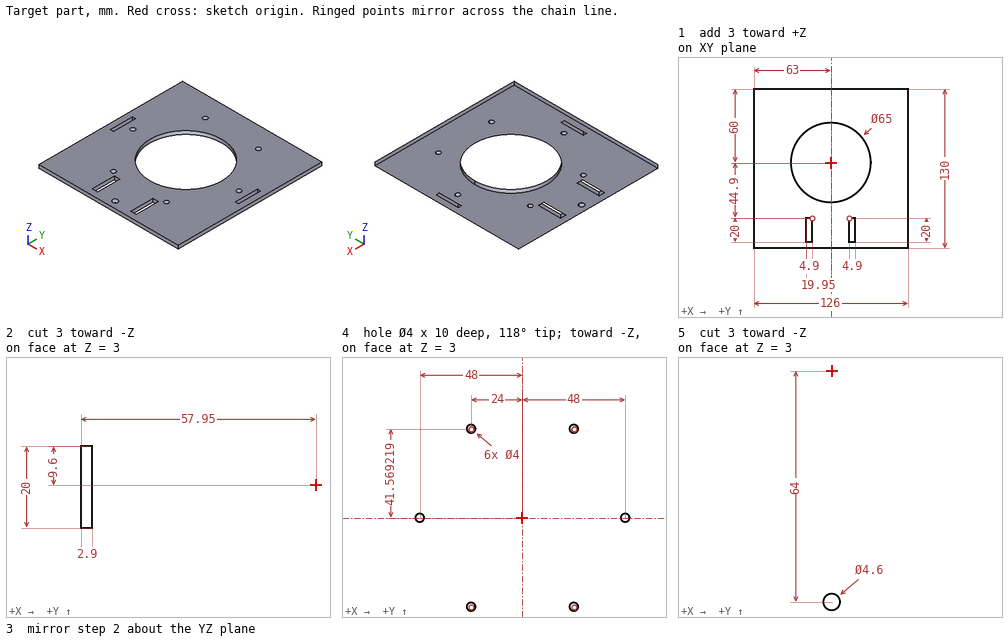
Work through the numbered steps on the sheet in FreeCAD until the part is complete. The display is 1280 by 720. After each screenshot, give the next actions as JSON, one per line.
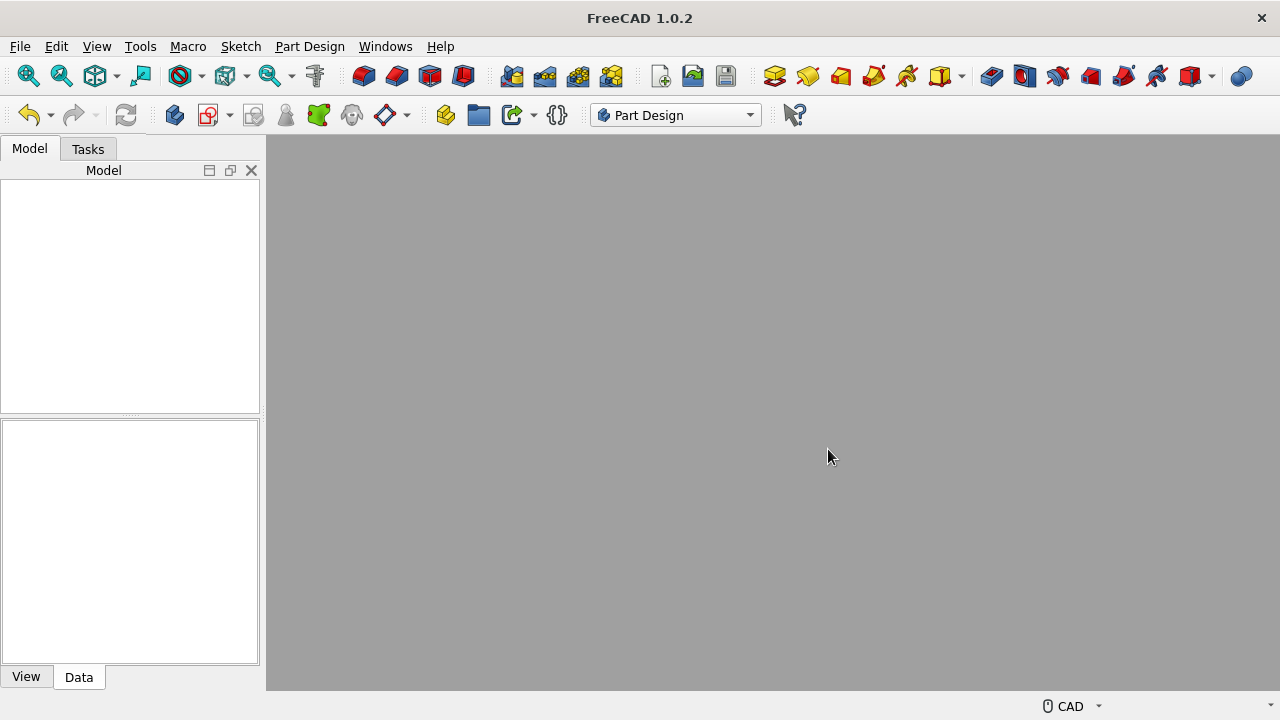
{"action": "left_click", "coordinate": [660, 76]}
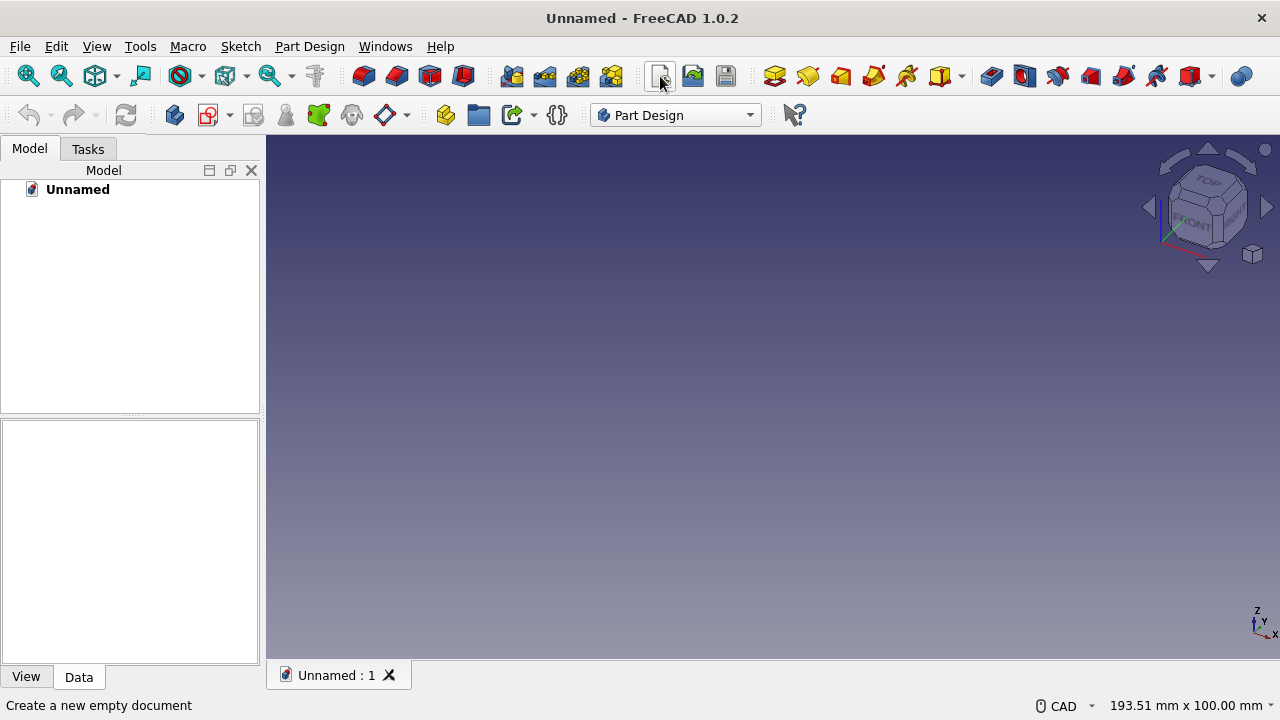
{"action": "left_click", "coordinate": [208, 116]}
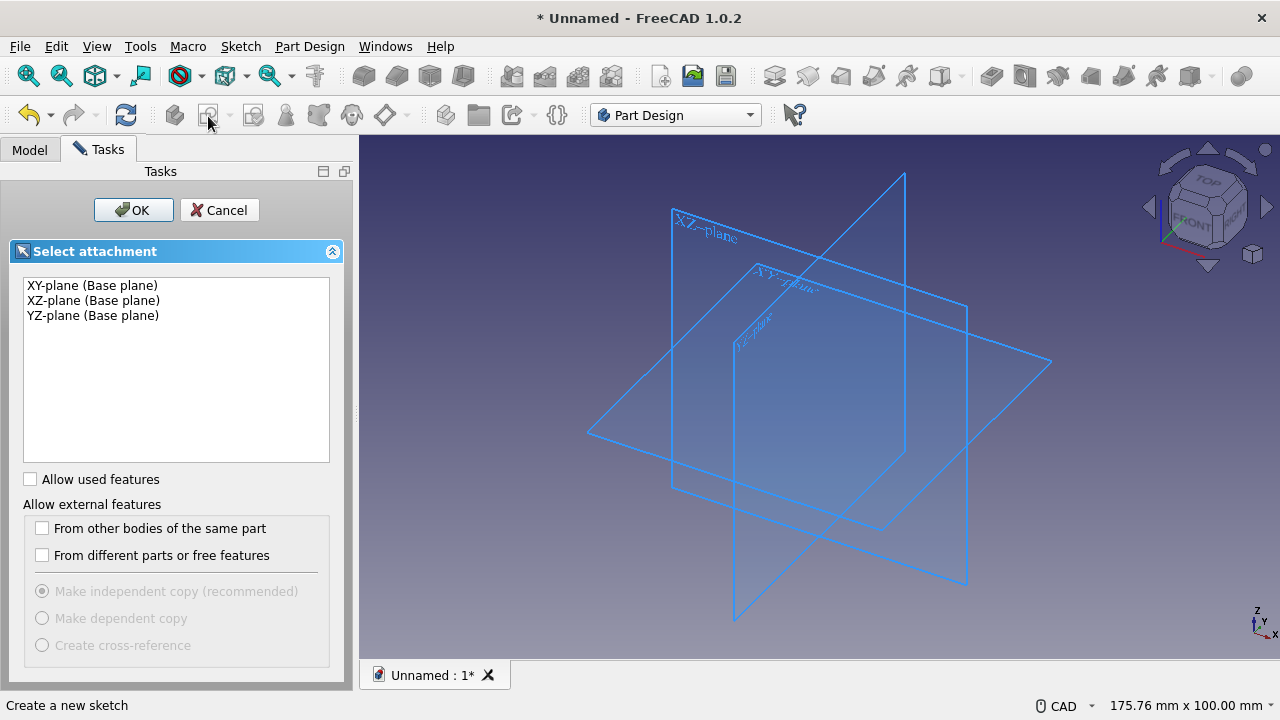
{"action": "left_click", "coordinate": [84, 286]}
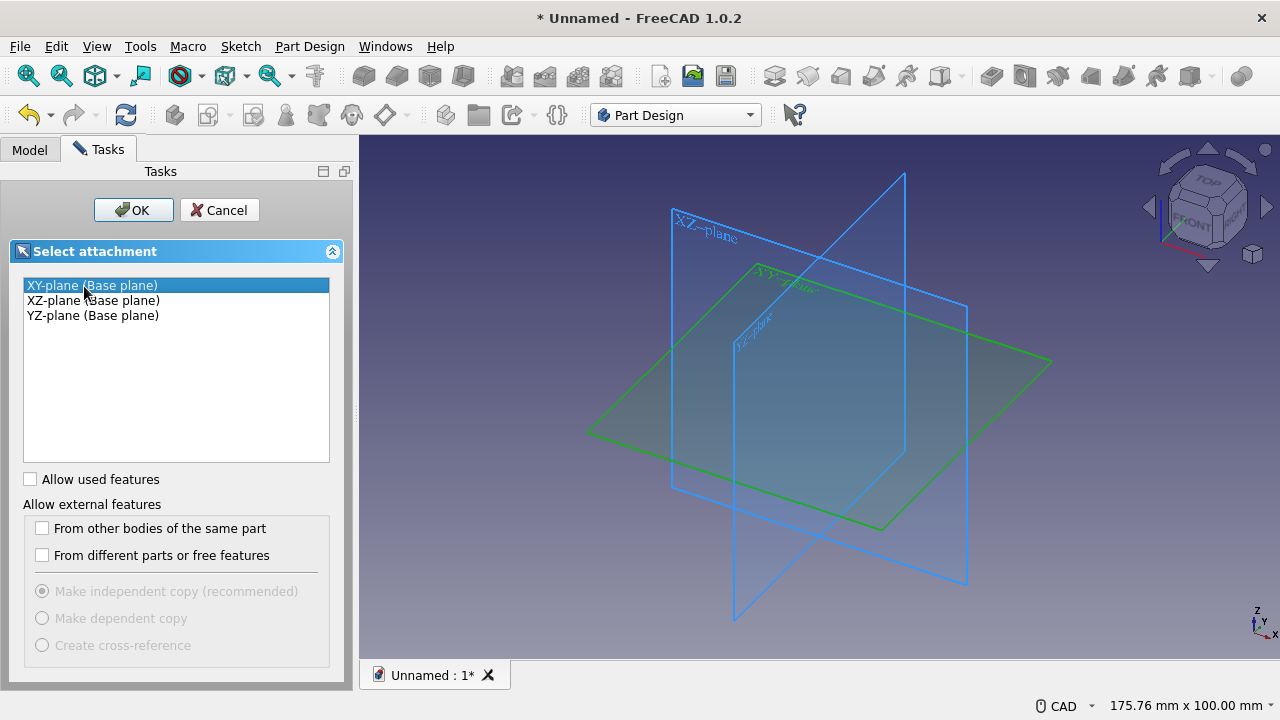
{"action": "left_click", "coordinate": [134, 210]}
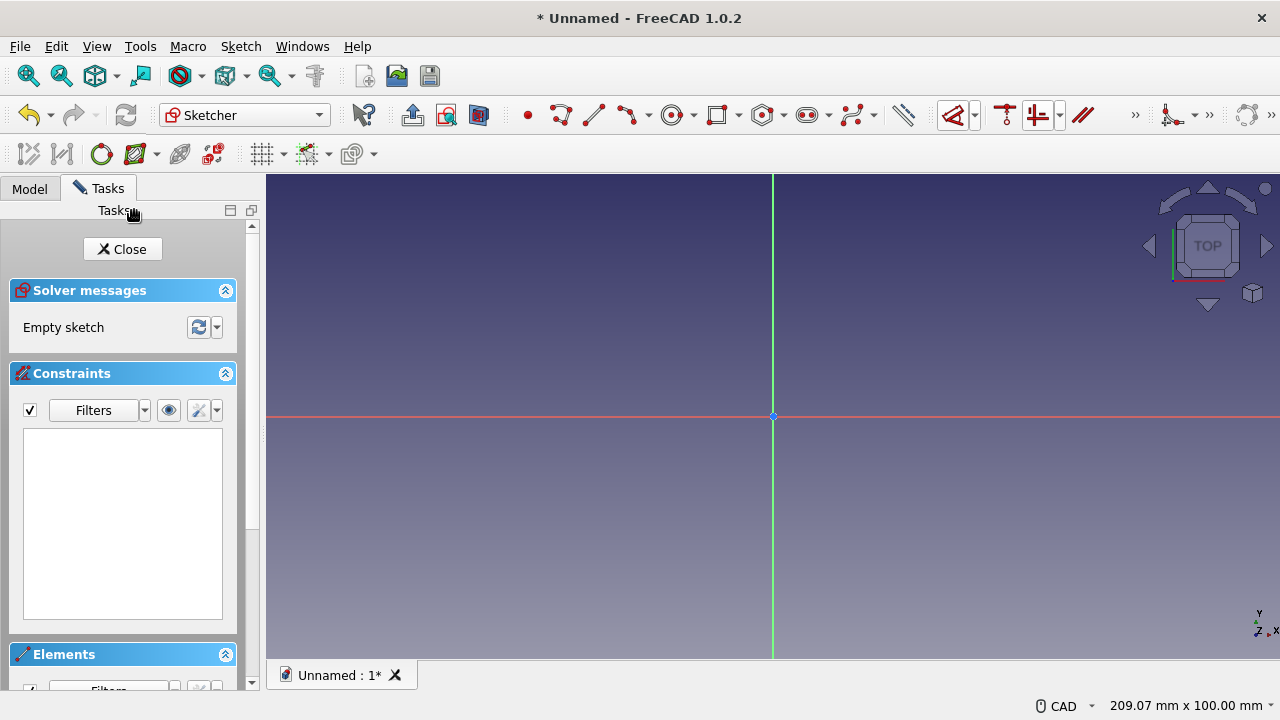
{"action": "scroll", "coordinate": [649, 397], "scroll_direction": "down", "scroll_amount": 4}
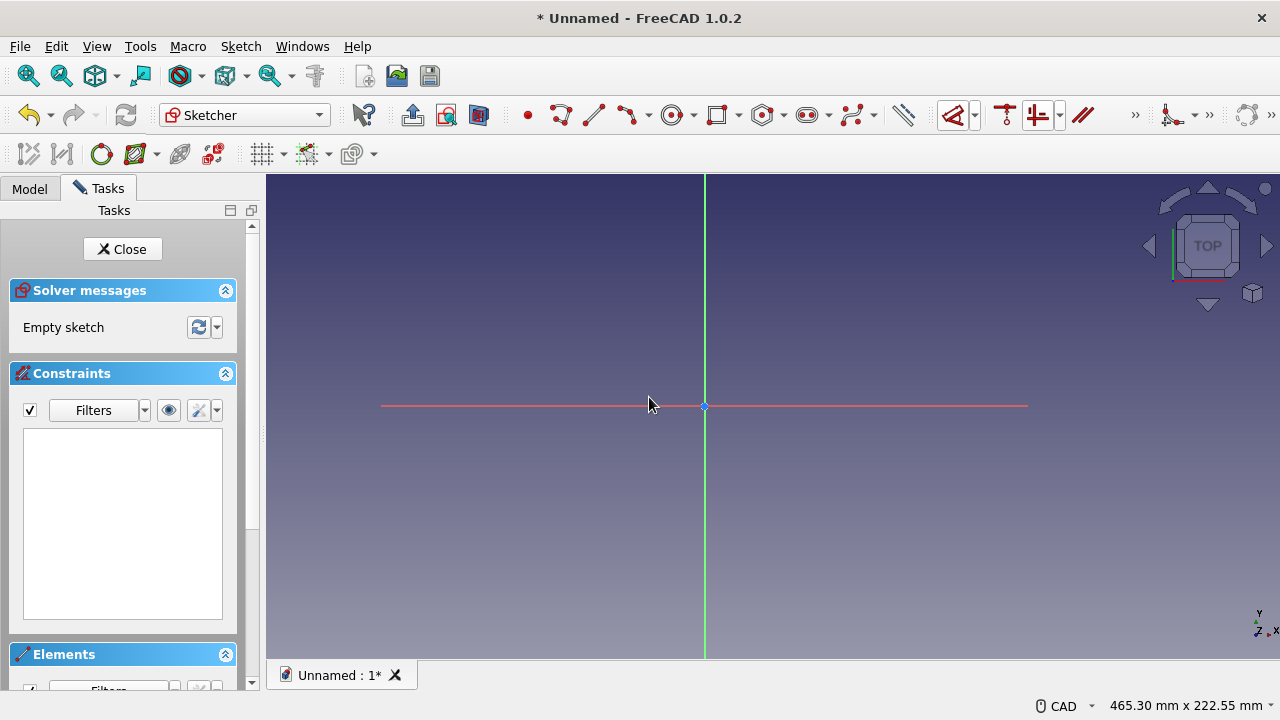
{"action": "left_click", "coordinate": [716, 116]}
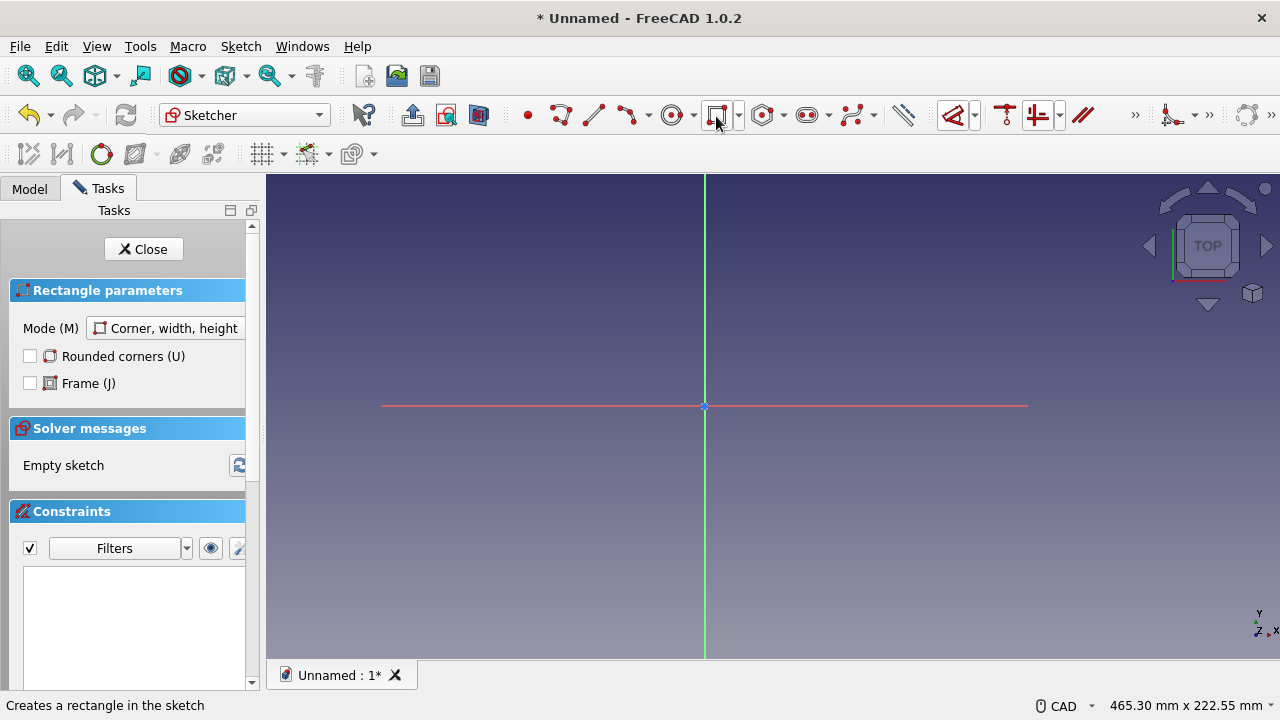
{"action": "left_click", "coordinate": [568, 275]}
{"action": "mouse_move", "coordinate": [842, 559]}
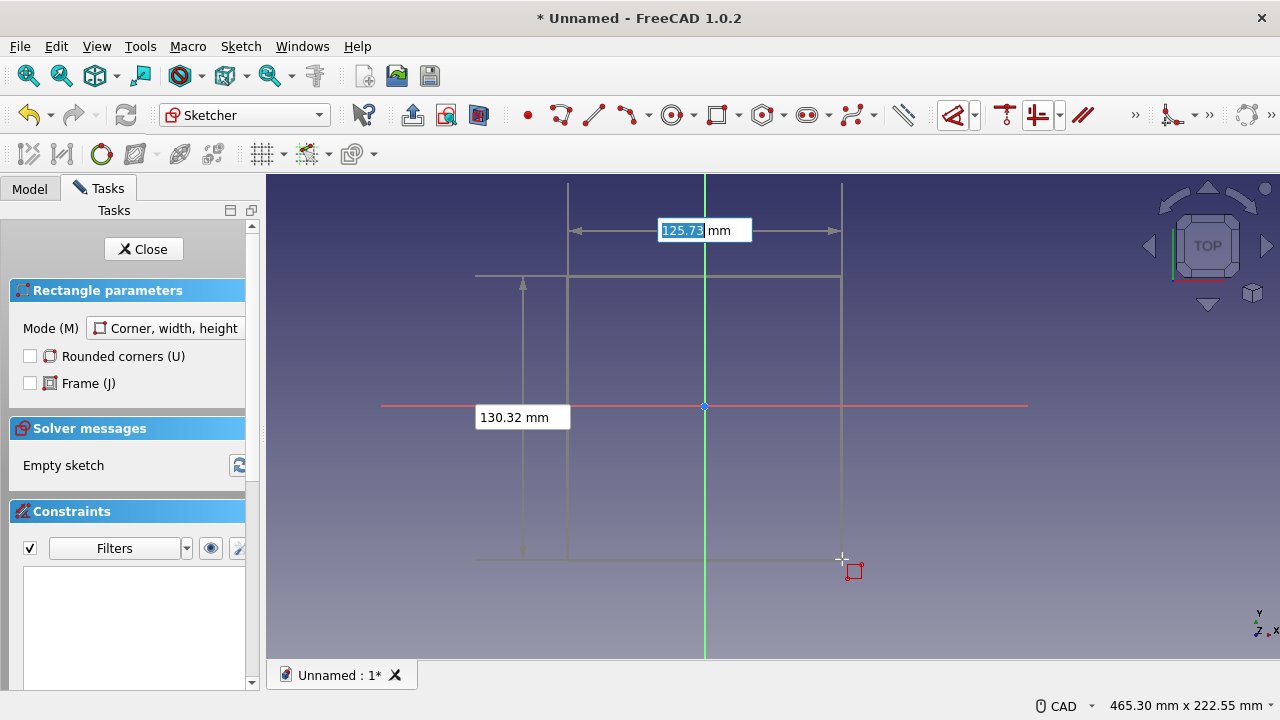
{"action": "type", "text": "126"}
{"action": "key", "text": "Tab"}
{"action": "type", "text": "130"}
{"action": "key", "text": "Return"}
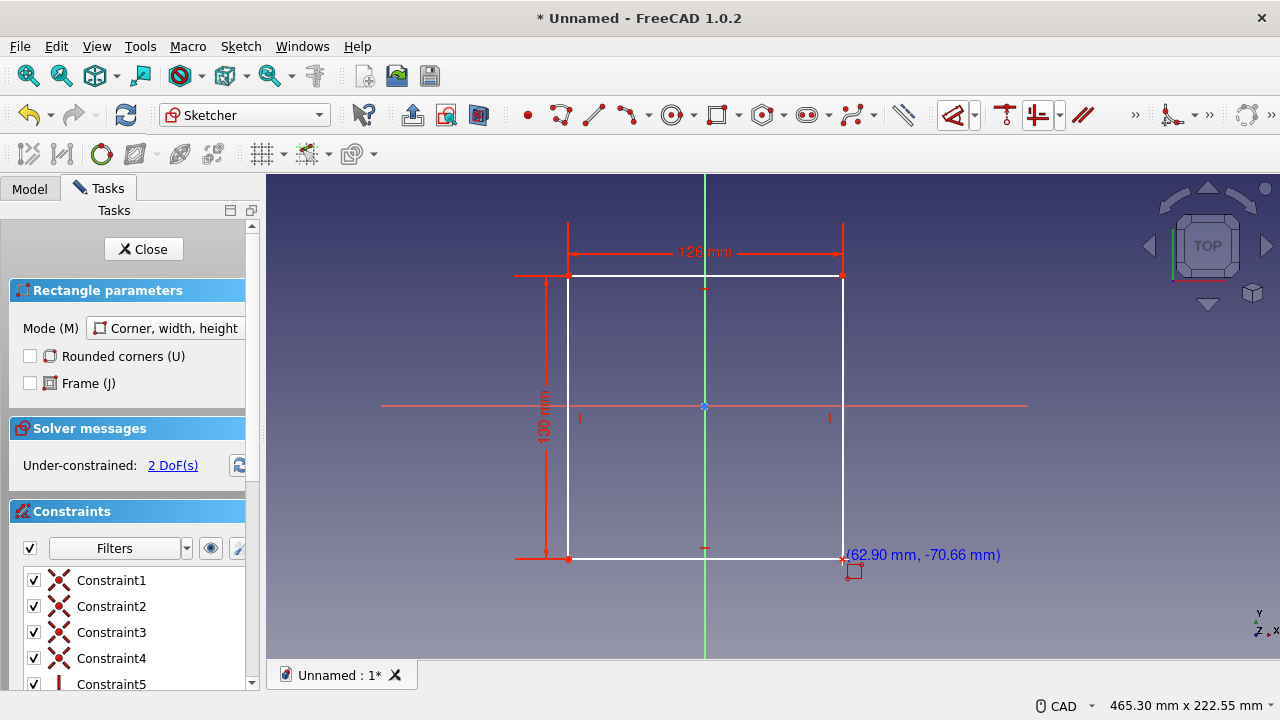
{"action": "scroll", "coordinate": [661, 504], "scroll_direction": "up", "scroll_amount": 2}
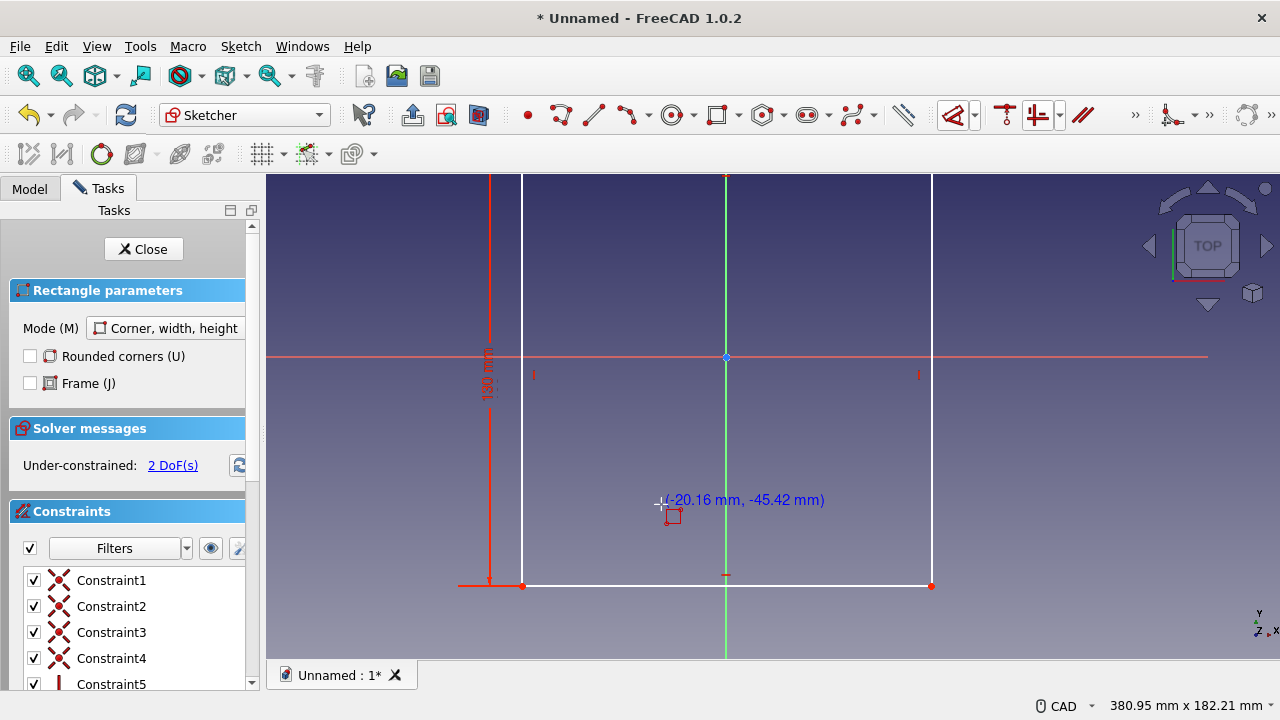
{"action": "left_click", "coordinate": [661, 503]}
{"action": "mouse_move", "coordinate": [677, 568]}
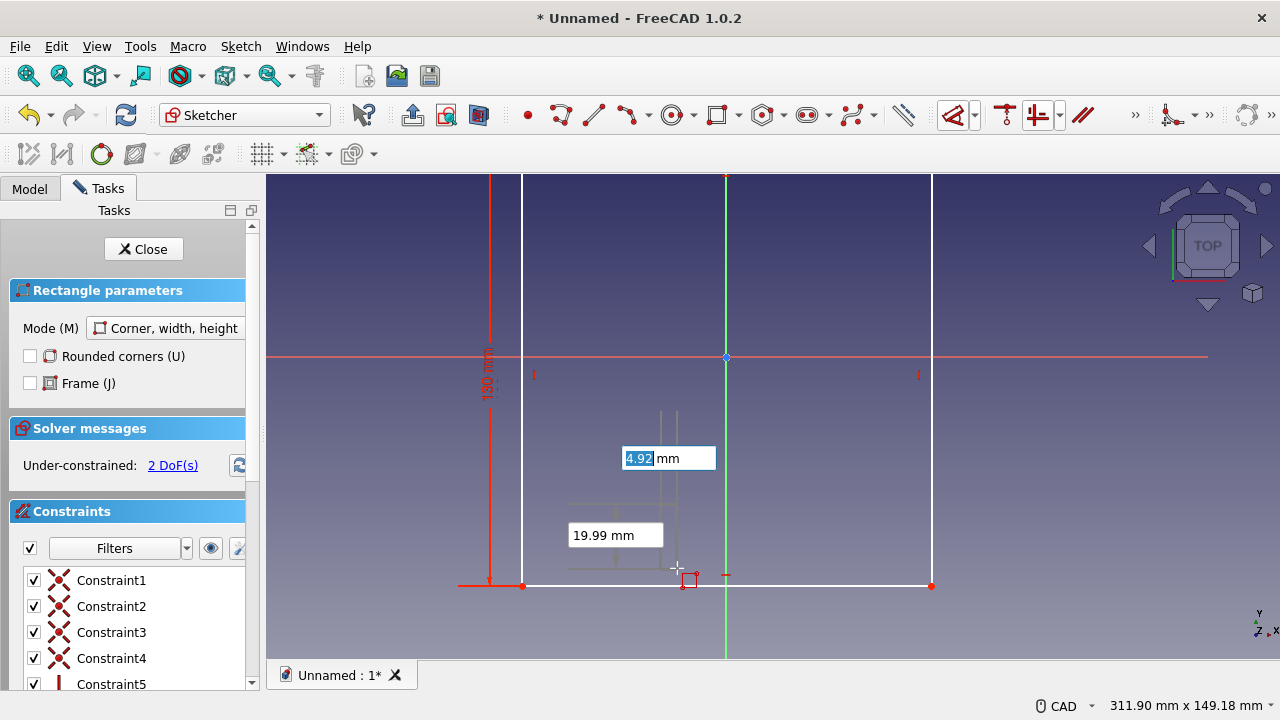
{"action": "type", "text": "4.9"}
{"action": "key", "text": "Tab"}
{"action": "type", "text": "20"}
{"action": "key", "text": "Return"}